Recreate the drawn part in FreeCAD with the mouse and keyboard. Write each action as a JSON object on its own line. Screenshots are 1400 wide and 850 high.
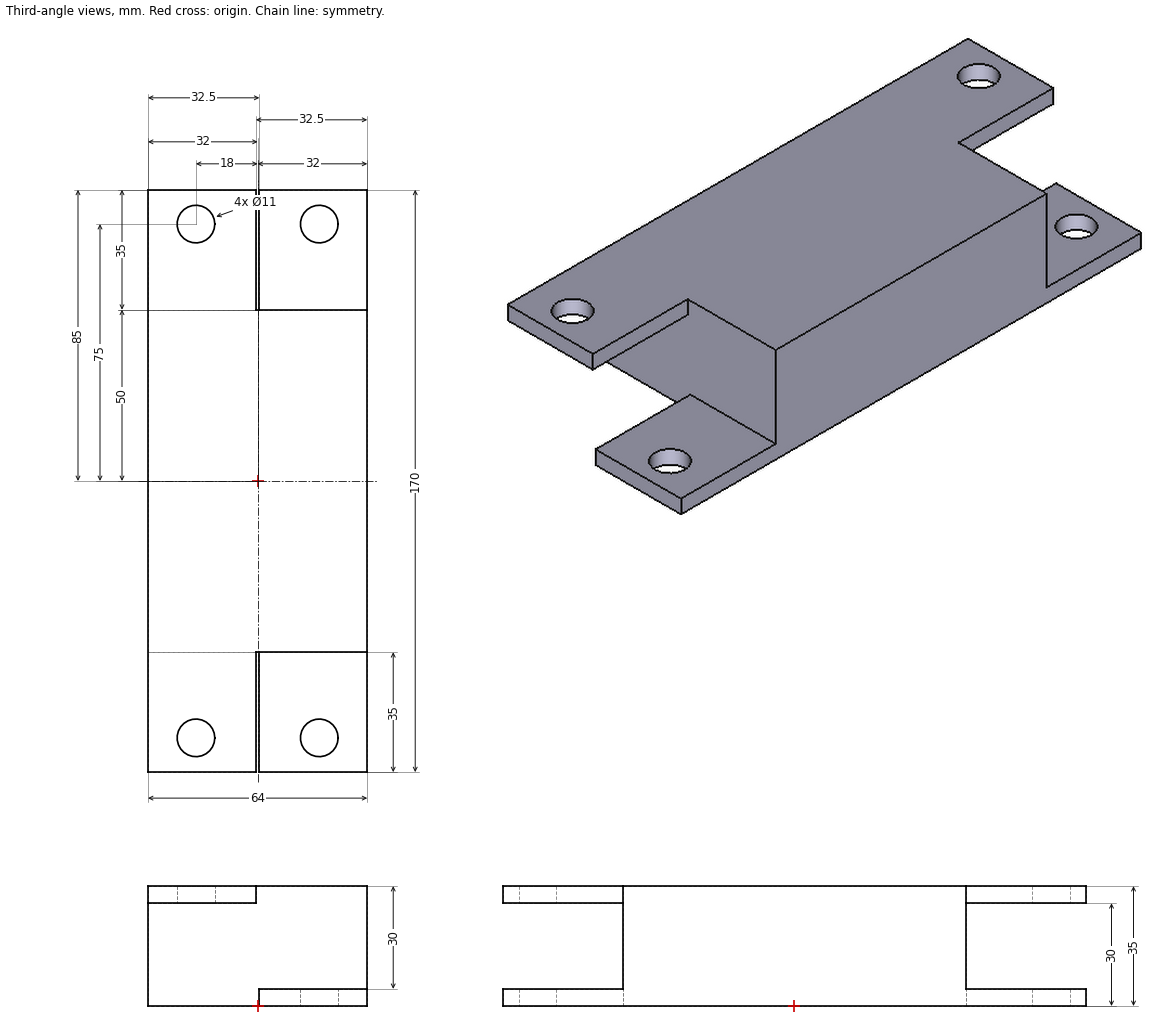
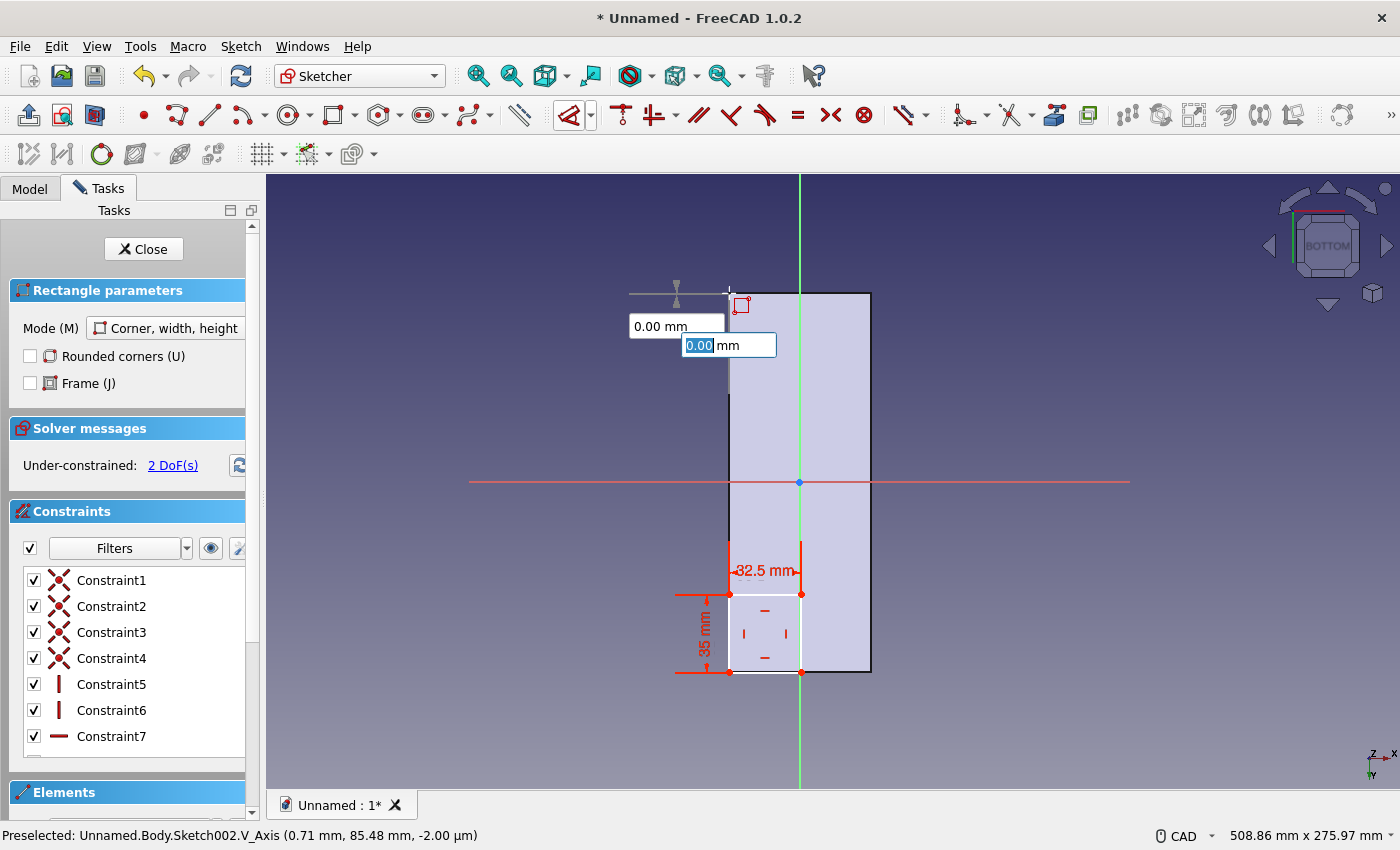
{"action": "scroll", "coordinate": [801, 371], "scroll_direction": "up", "scroll_amount": 14}
{"action": "mouse_move", "coordinate": [793, 366]}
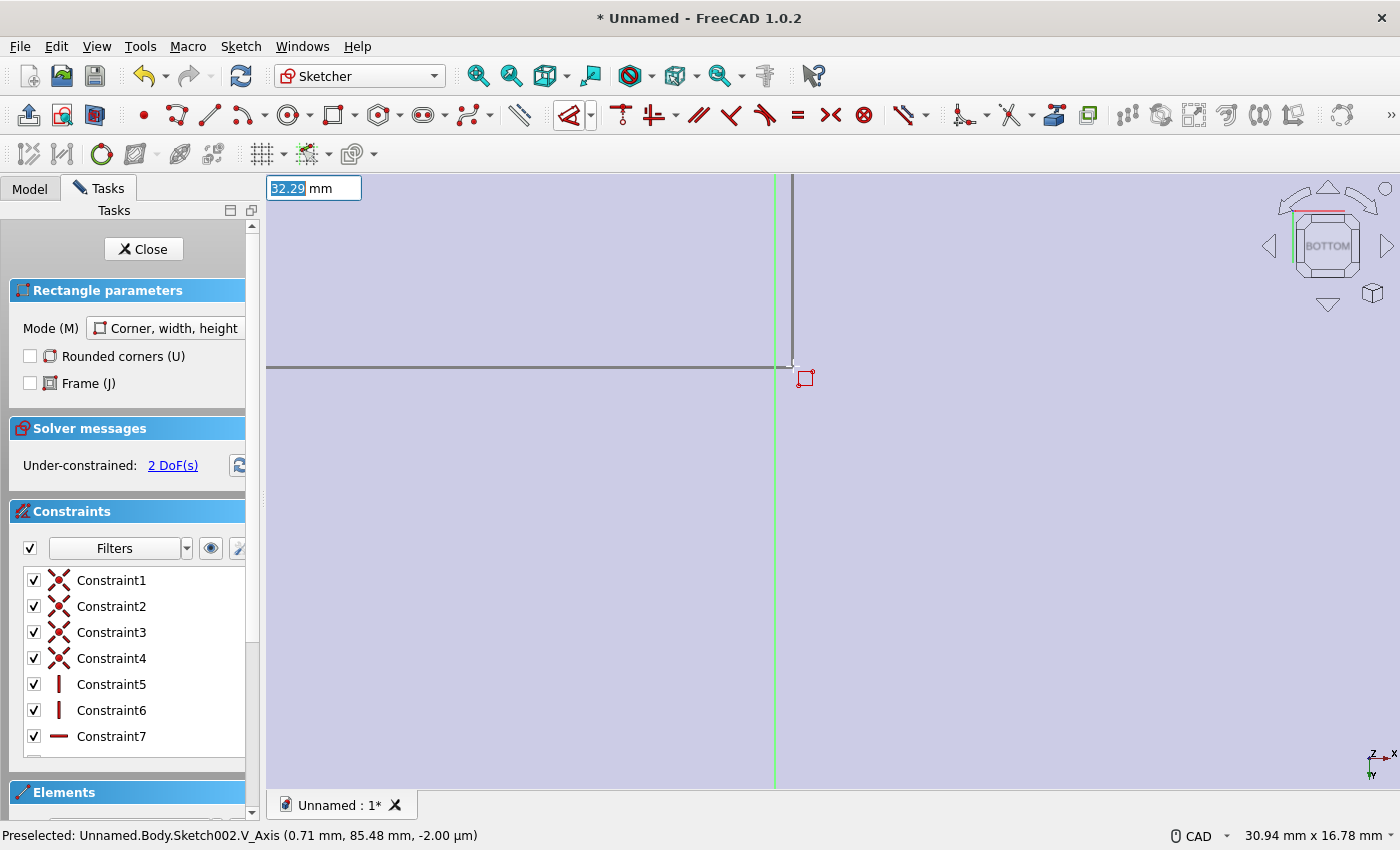
{"action": "type", "text": "32.5"}
{"action": "key", "text": "Tab"}
{"action": "type", "text": "35"}
{"action": "key", "text": "Return"}
{"action": "key", "text": "Escape"}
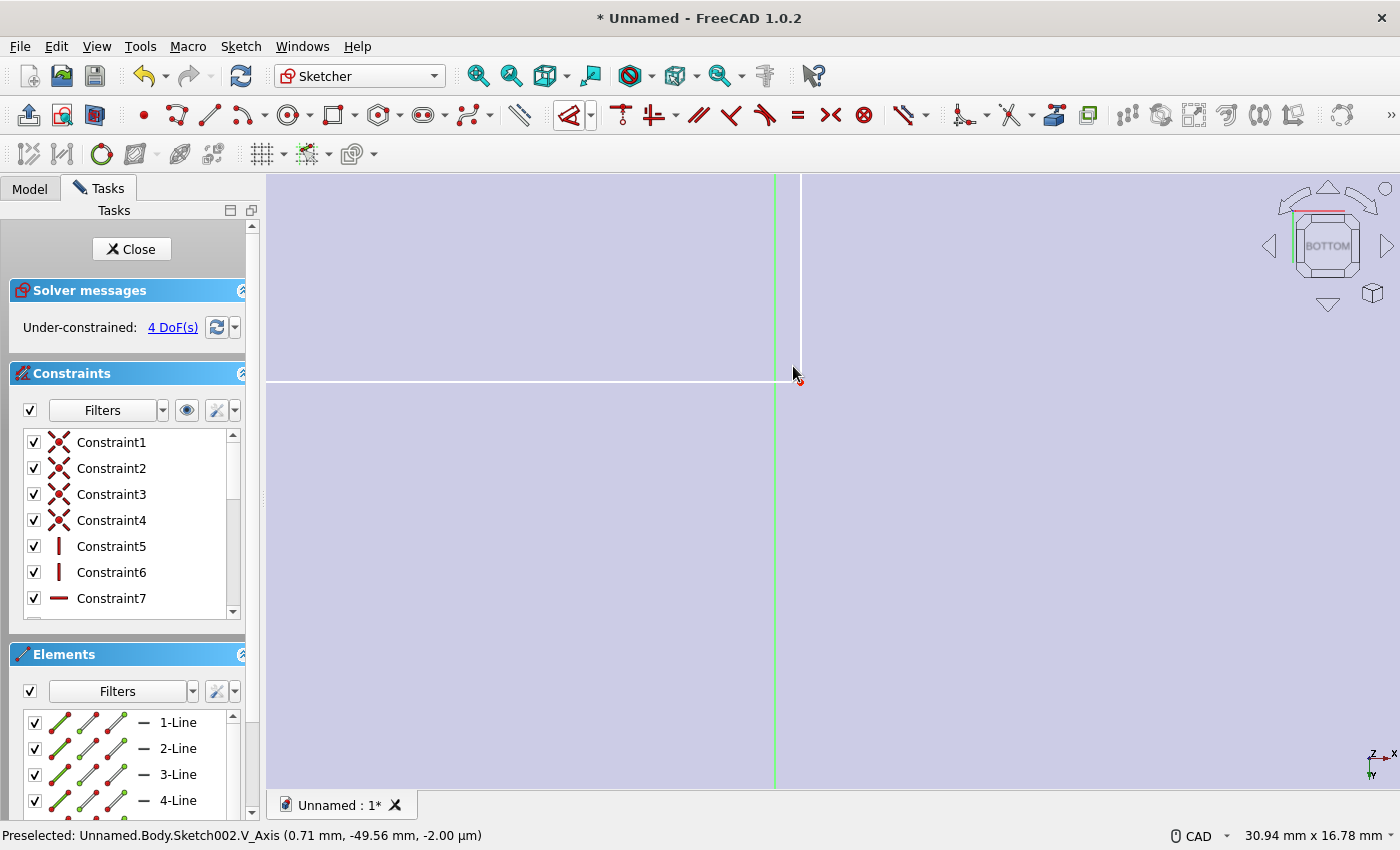
{"action": "scroll", "coordinate": [801, 370], "scroll_direction": "down", "scroll_amount": 14}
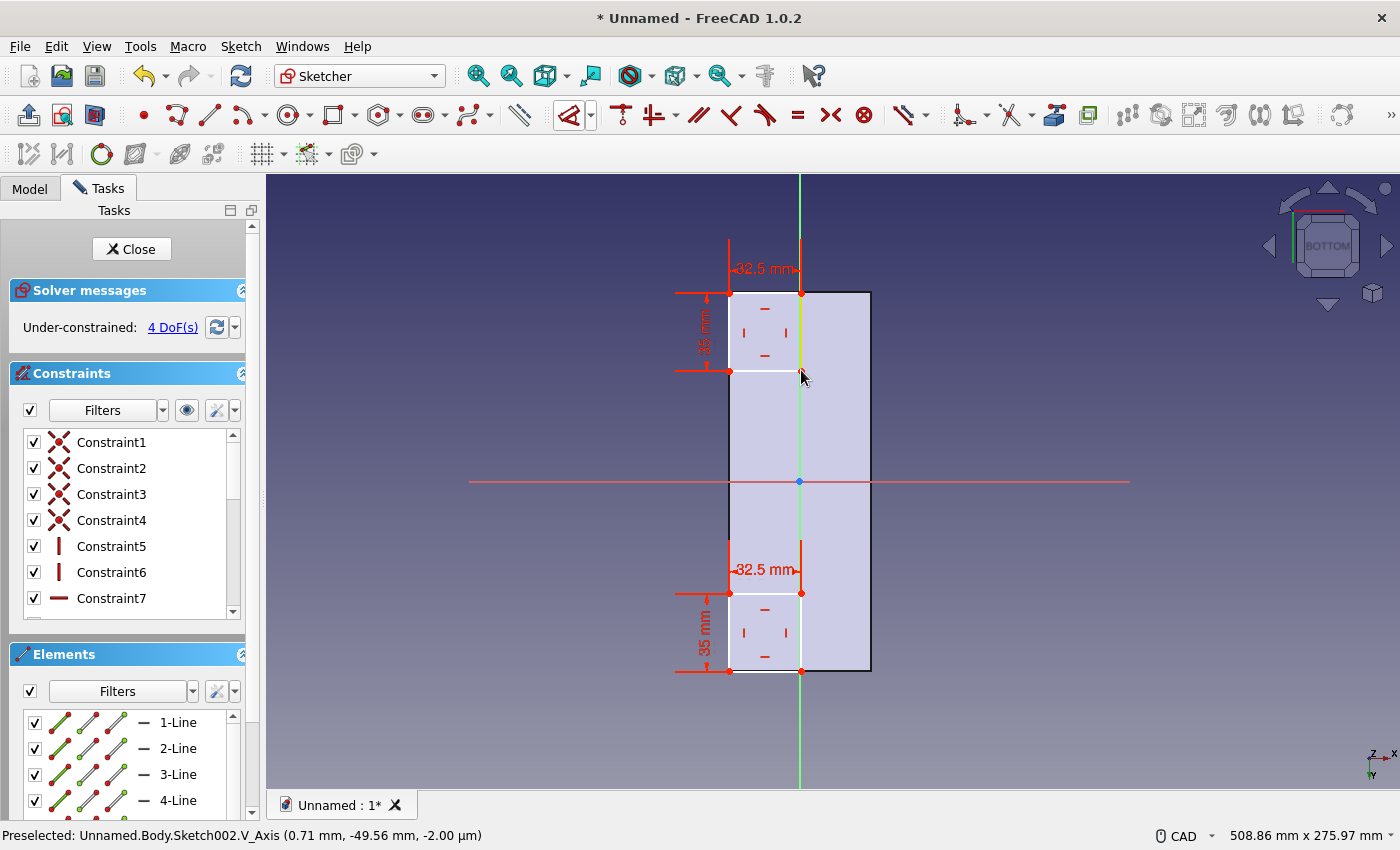
{"action": "left_click", "coordinate": [729, 672]}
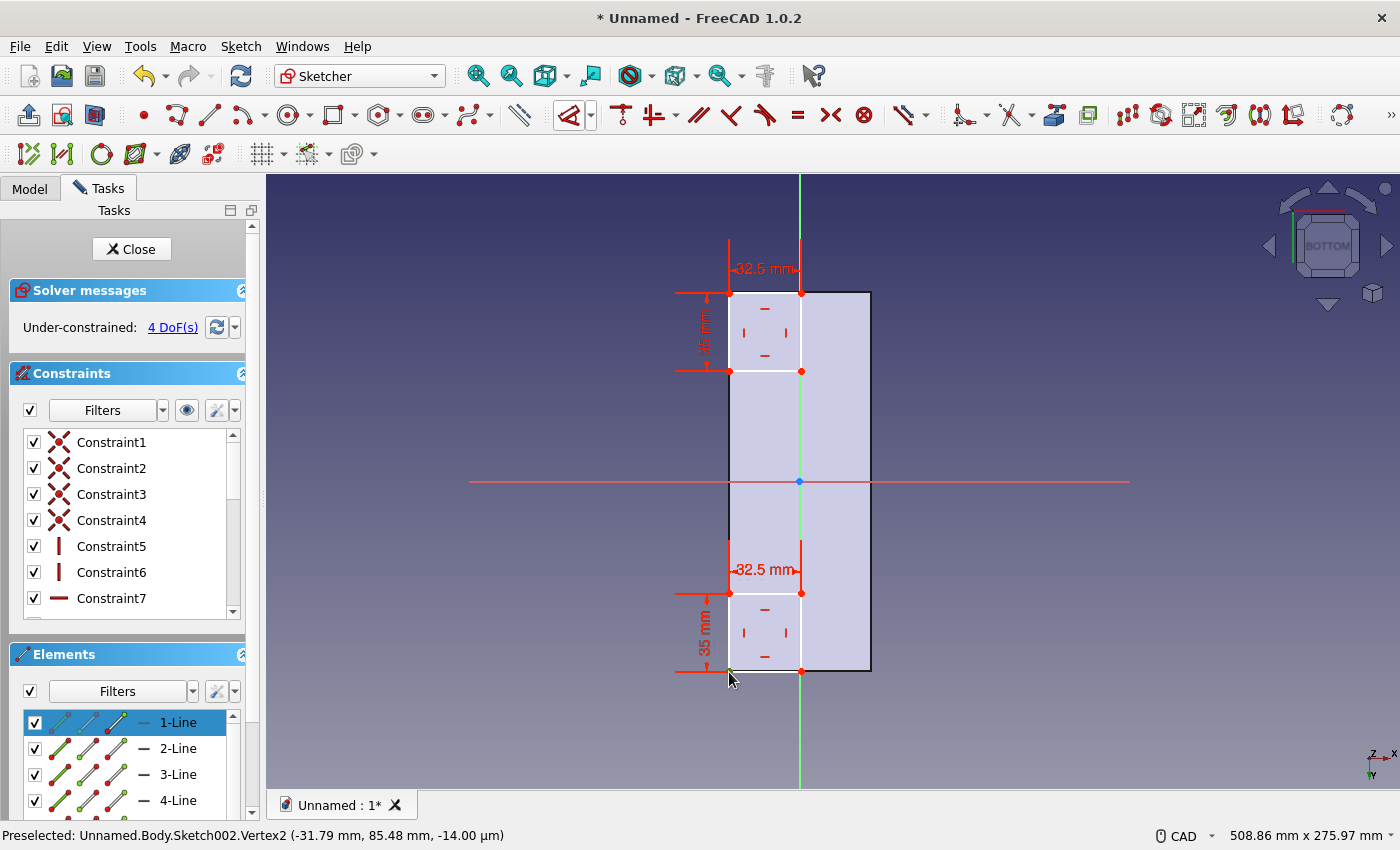
{"action": "left_click", "coordinate": [729, 293]}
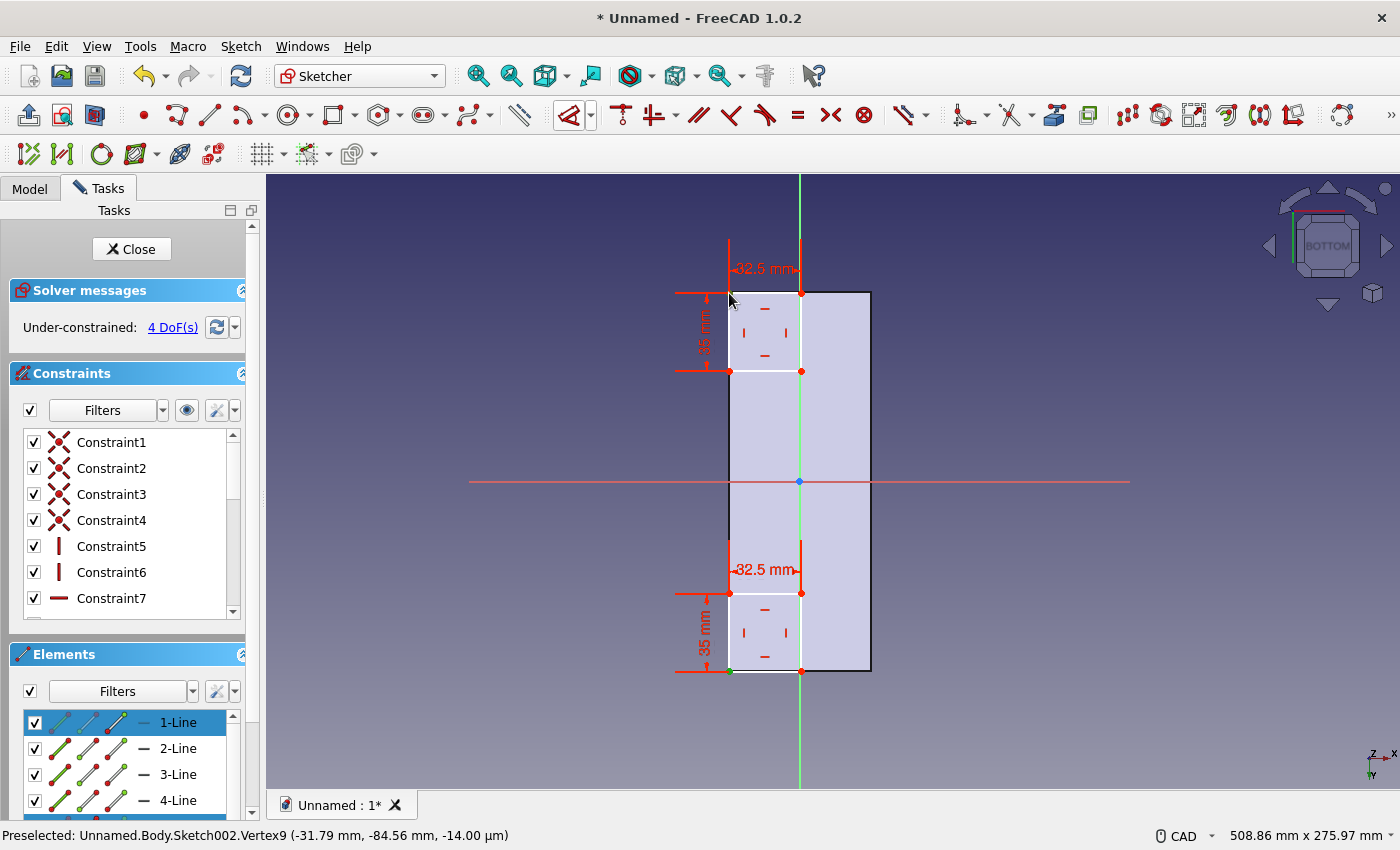
{"action": "left_click", "coordinate": [496, 481]}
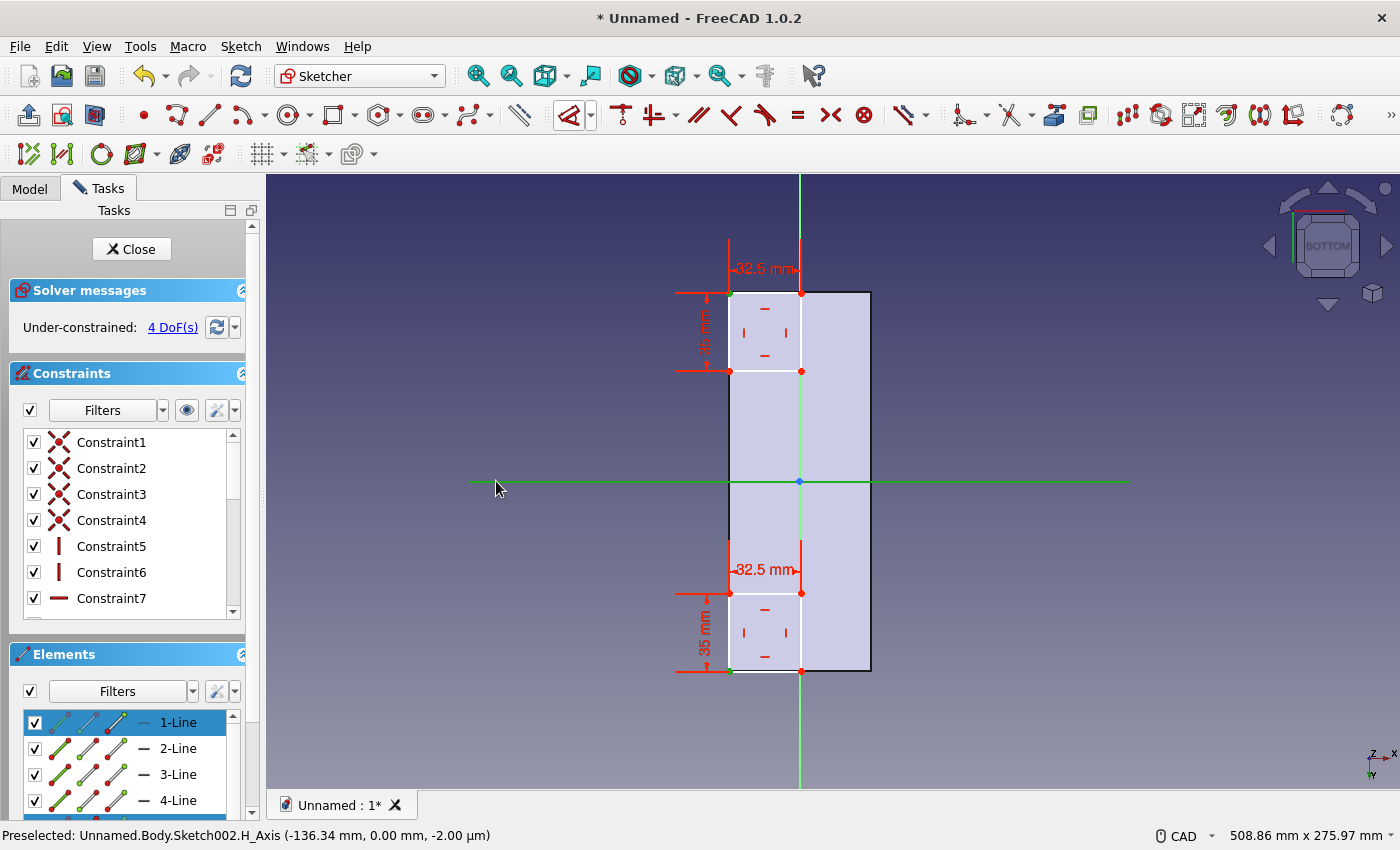
{"action": "left_click", "coordinate": [831, 116]}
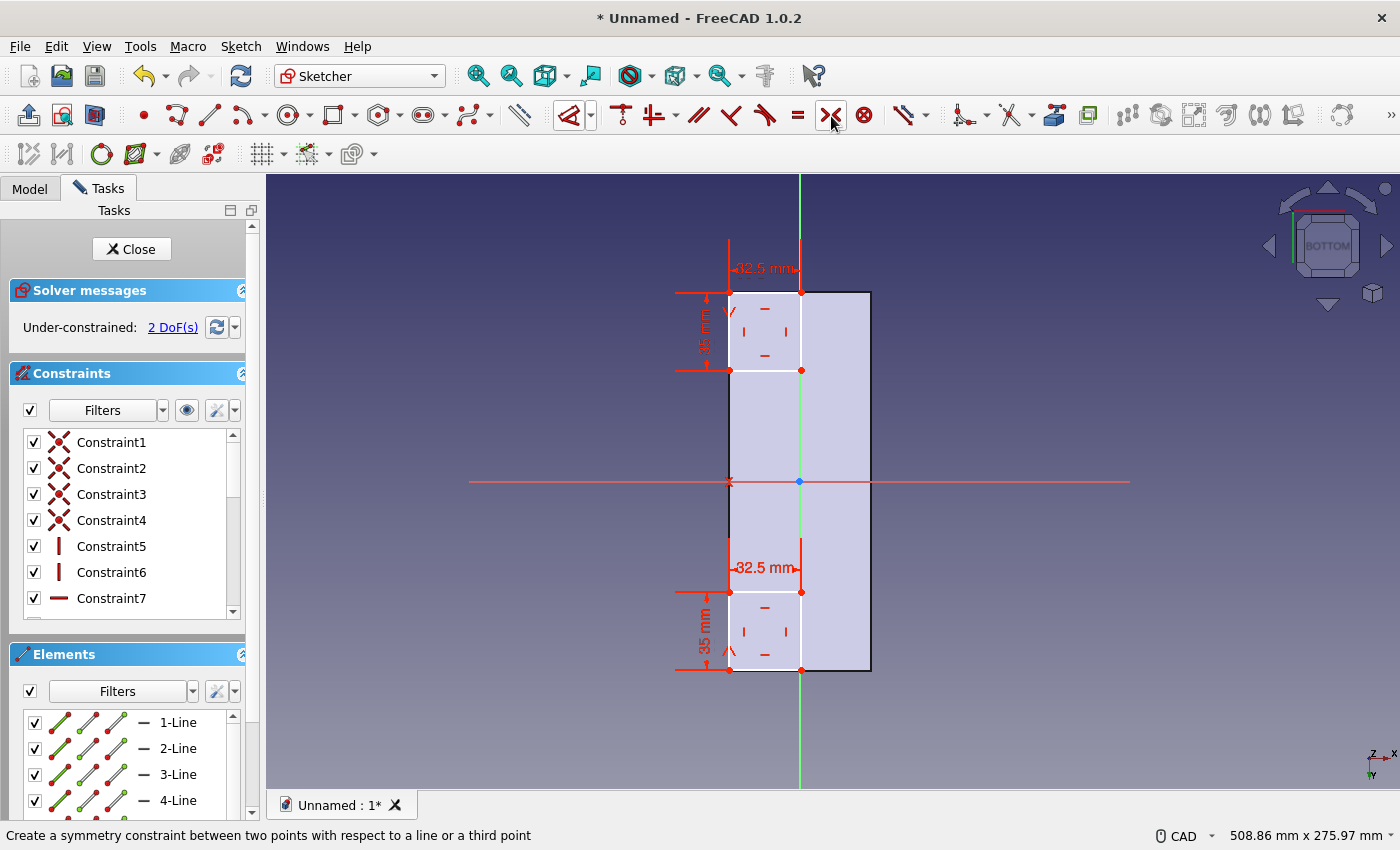
{"action": "left_click", "coordinate": [729, 592]}